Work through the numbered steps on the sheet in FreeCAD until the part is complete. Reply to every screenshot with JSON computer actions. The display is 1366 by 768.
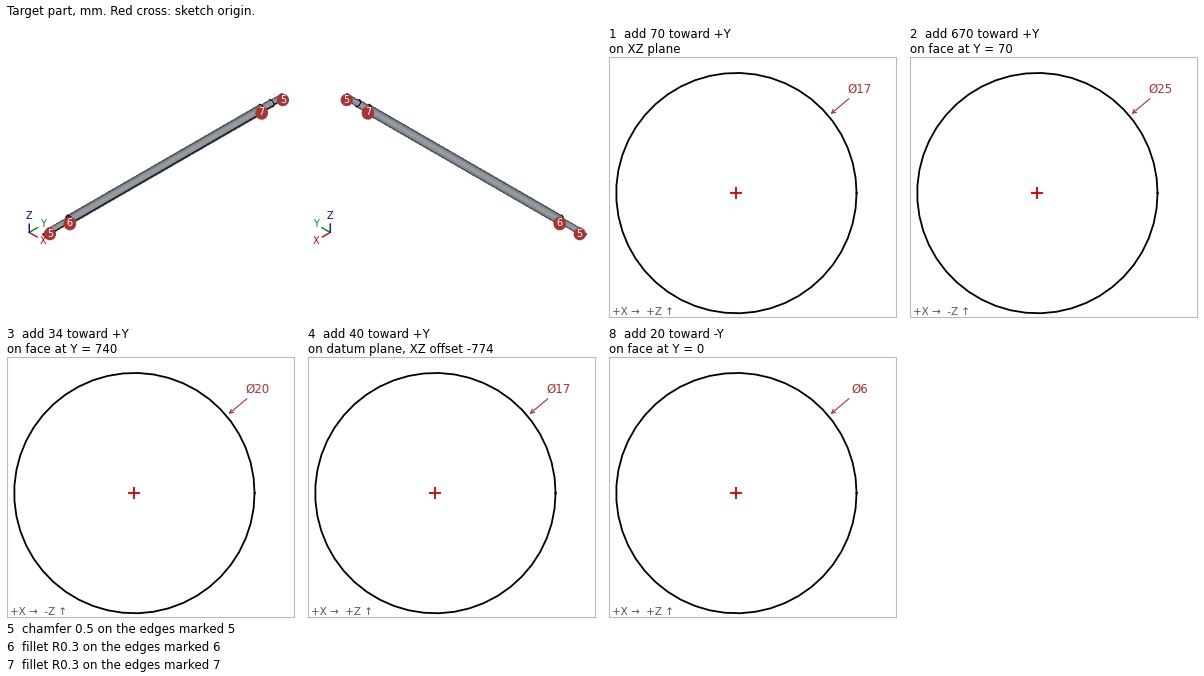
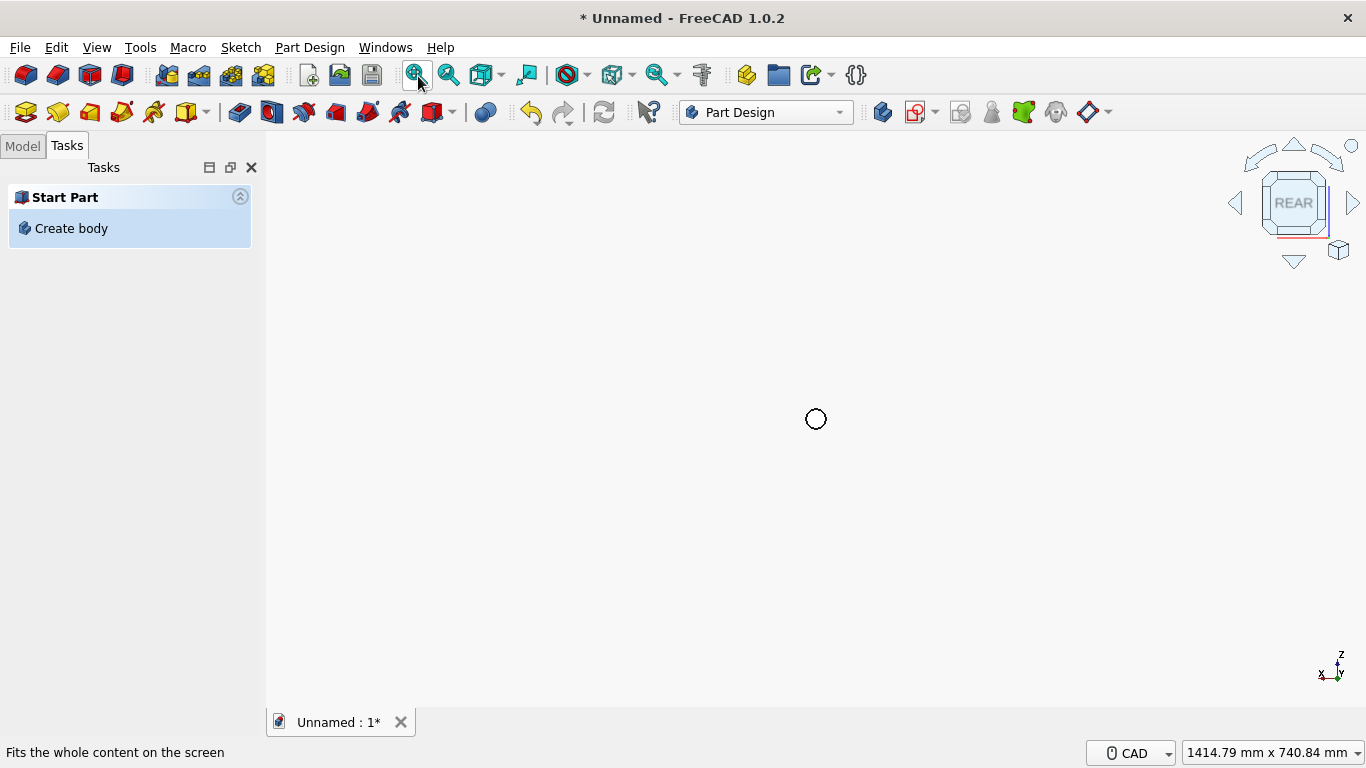
{"action": "left_click", "coordinate": [816, 418]}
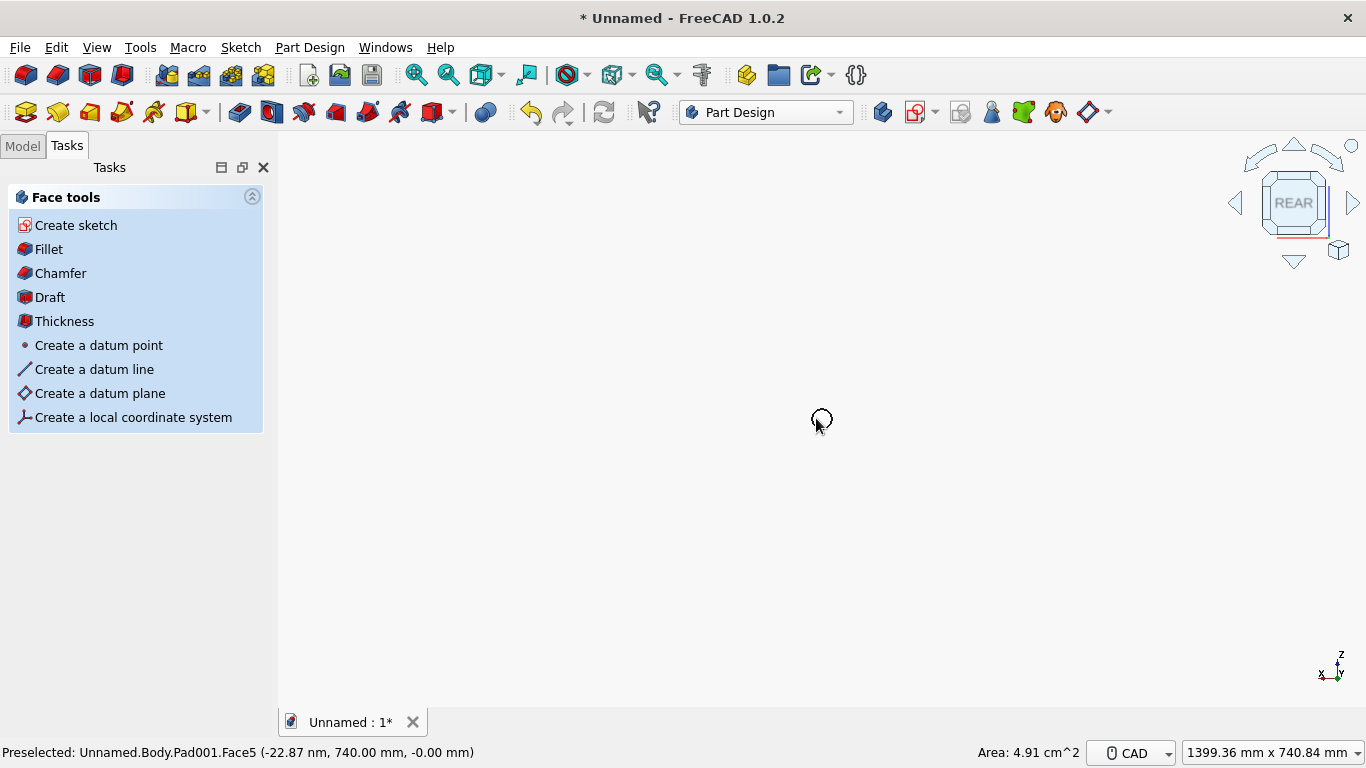
{"action": "left_click", "coordinate": [916, 112]}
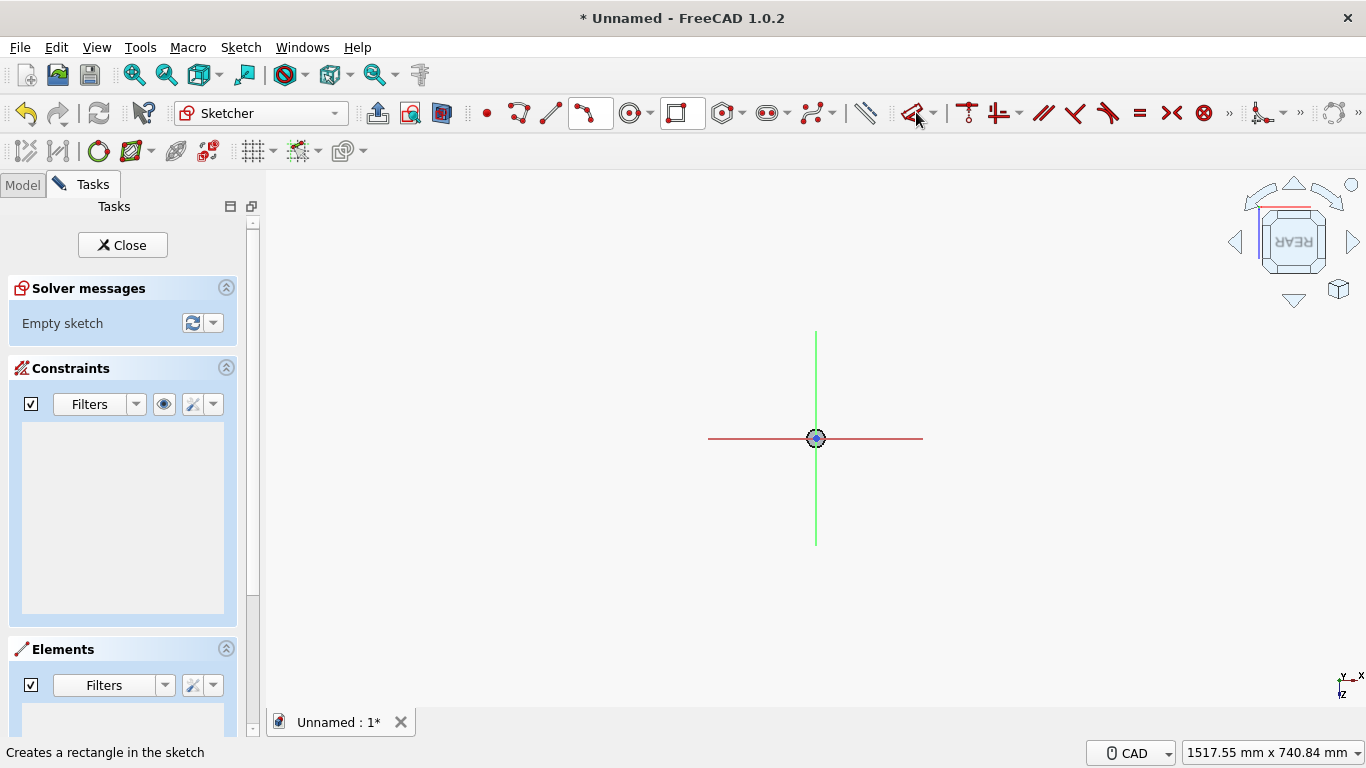
{"action": "scroll", "coordinate": [820, 438], "scroll_direction": "up", "scroll_amount": 15}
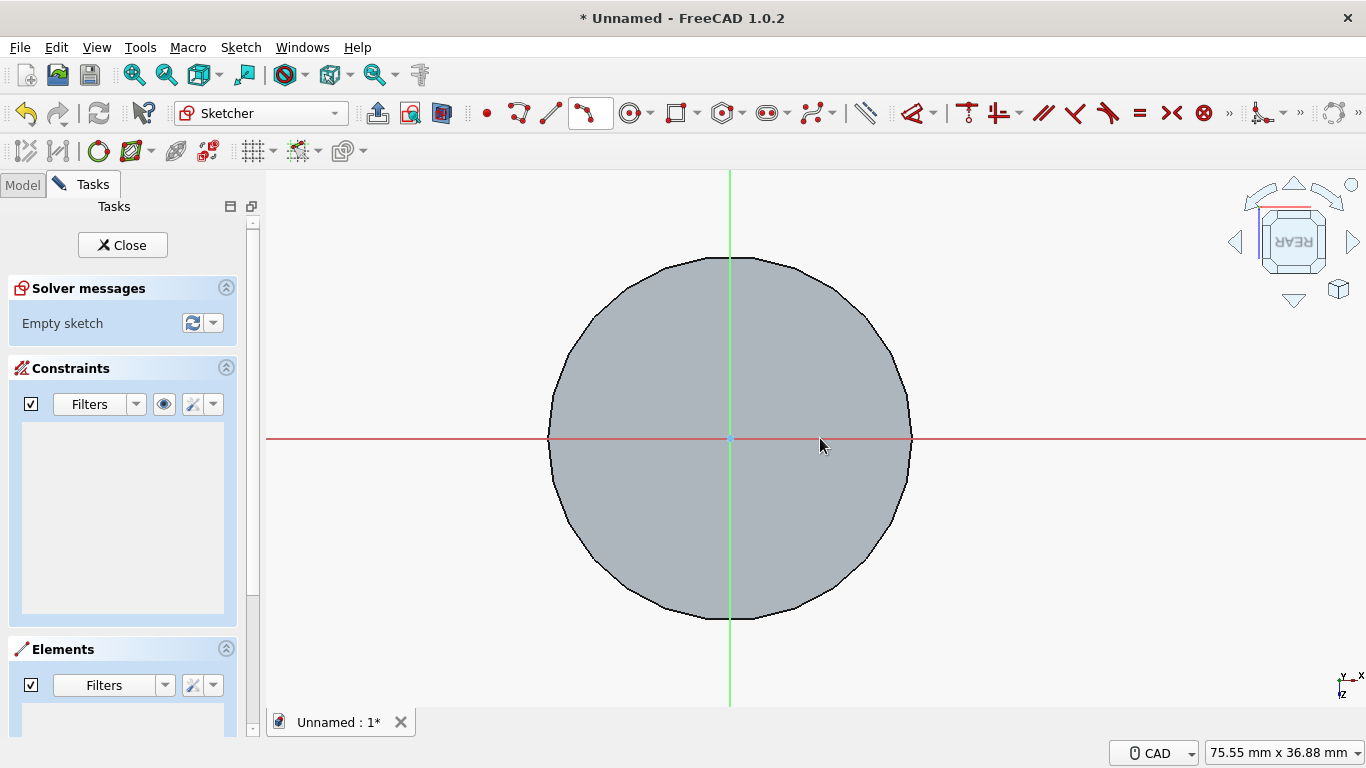
{"action": "left_click", "coordinate": [630, 114]}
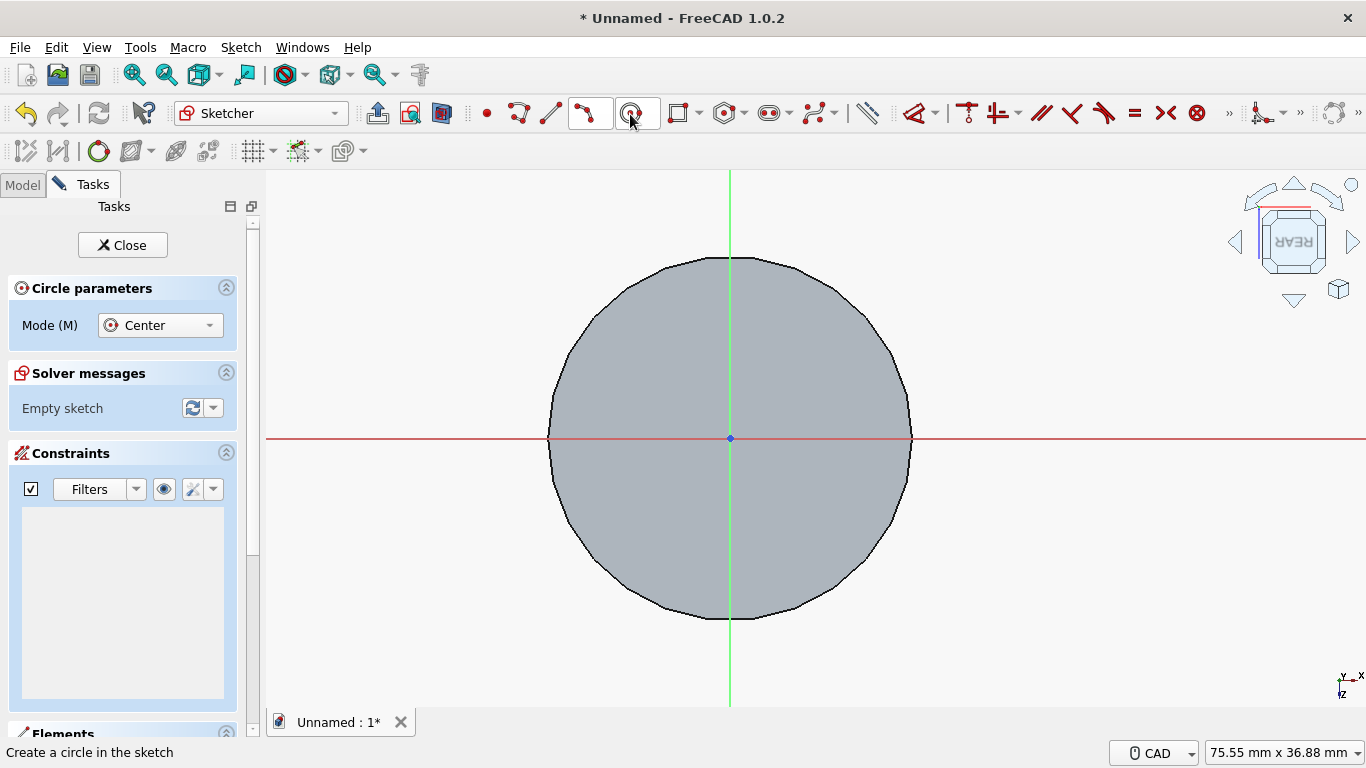
{"action": "left_click", "coordinate": [730, 438]}
{"action": "left_click", "coordinate": [833, 336]}
{"action": "key", "text": "Escape"}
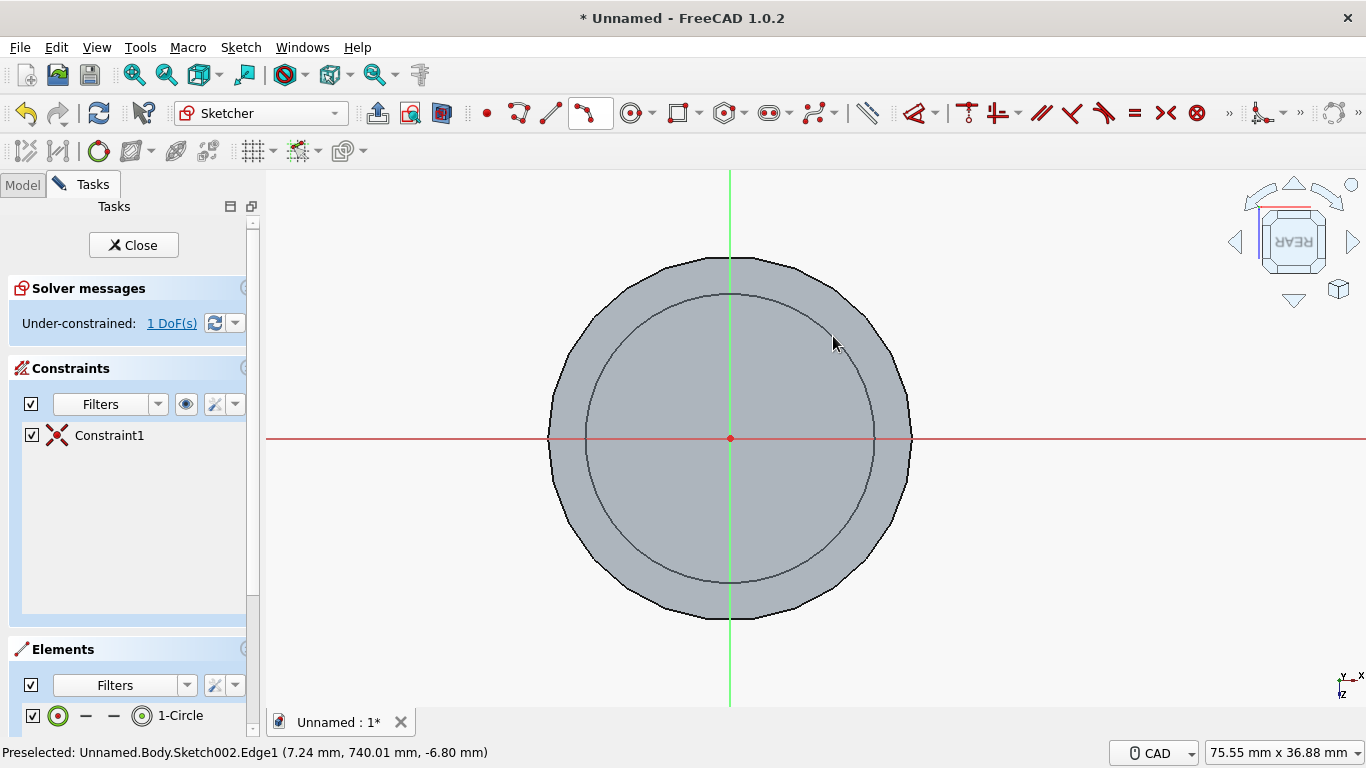
{"action": "key", "text": "d"}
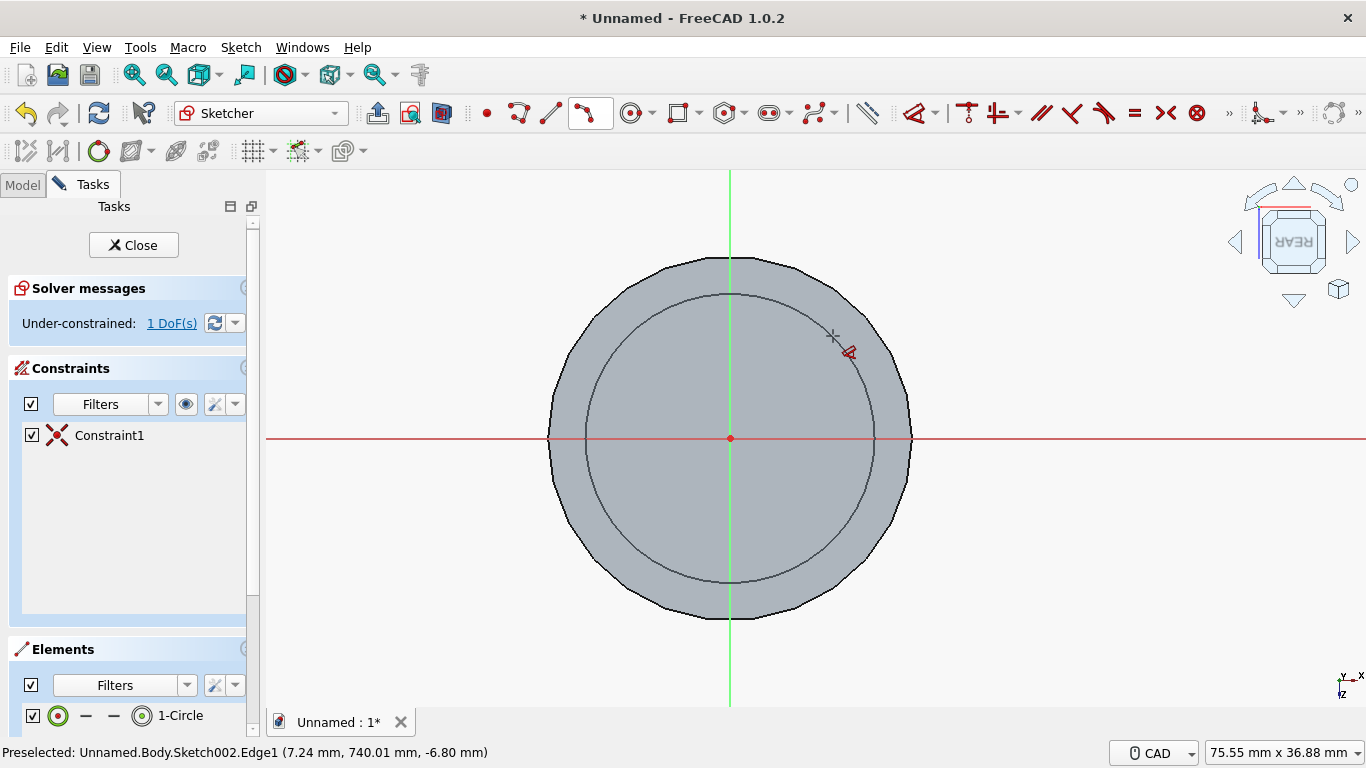
{"action": "left_click", "coordinate": [832, 336]}
{"action": "left_click", "coordinate": [855, 313]}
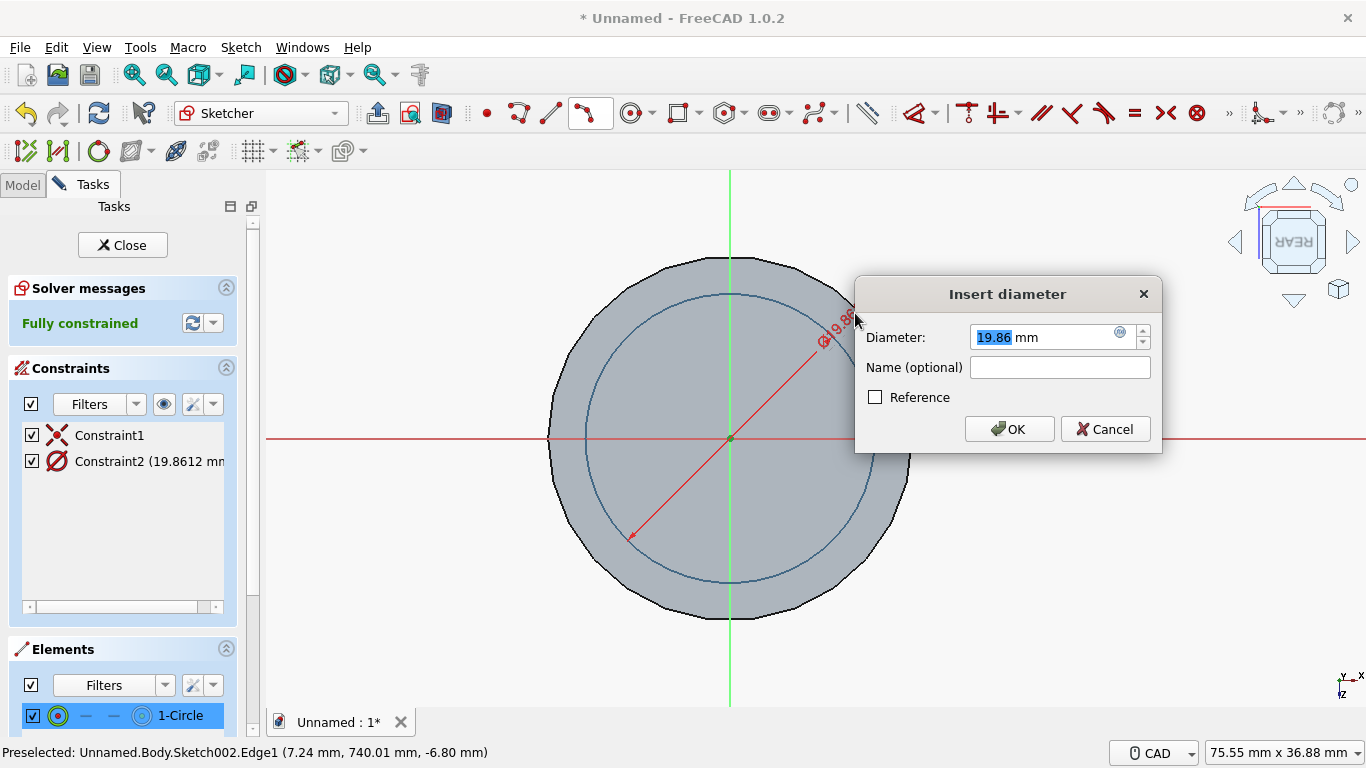
{"action": "type", "text": "20"}
{"action": "key", "text": "Return"}
{"action": "key", "text": "Escape"}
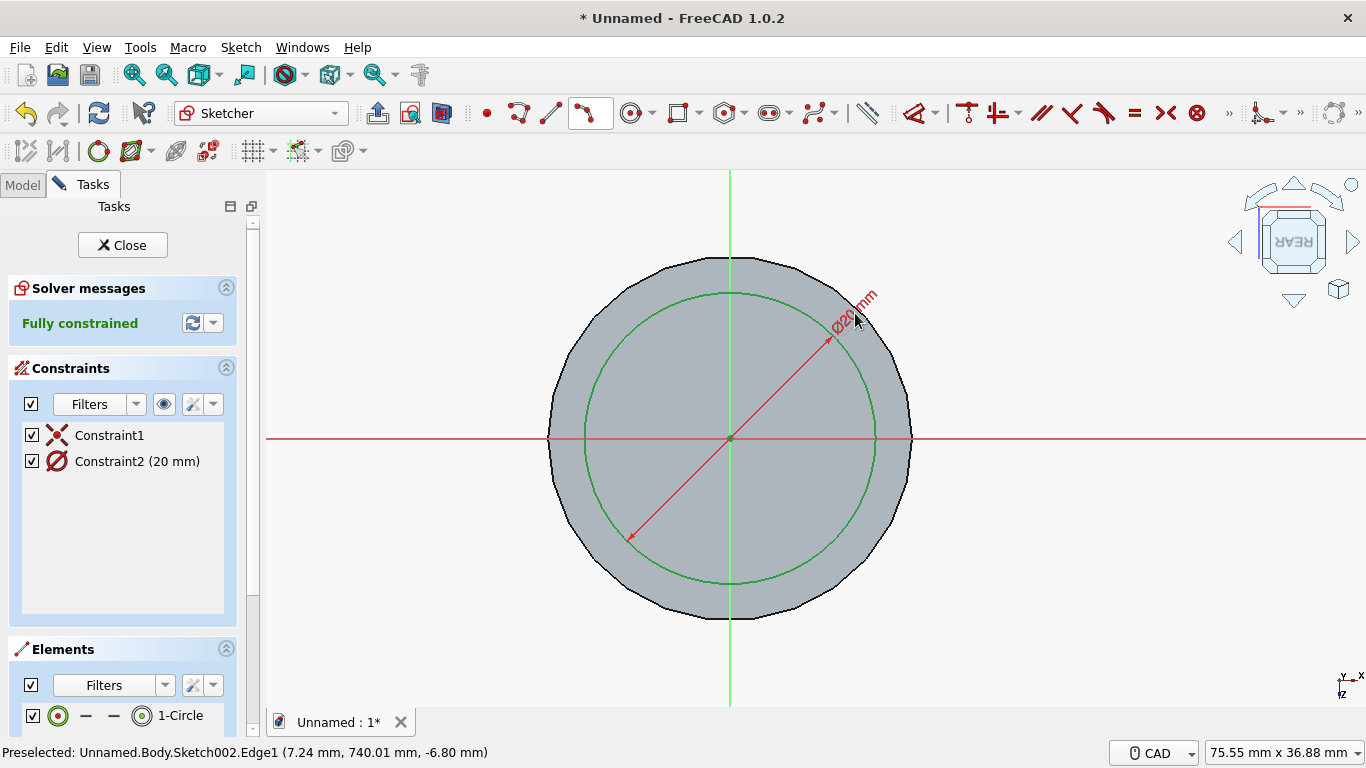
{"action": "left_click", "coordinate": [123, 245]}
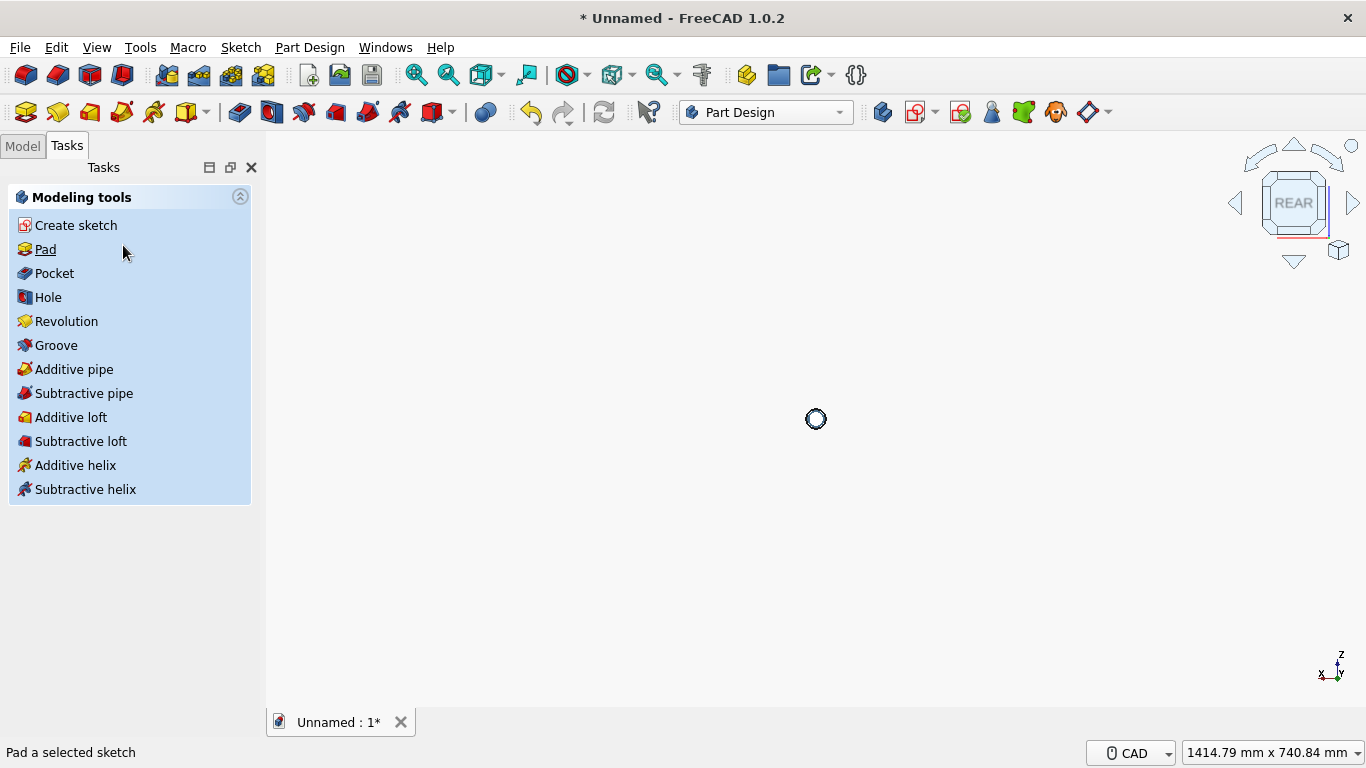
{"action": "left_click", "coordinate": [26, 112]}